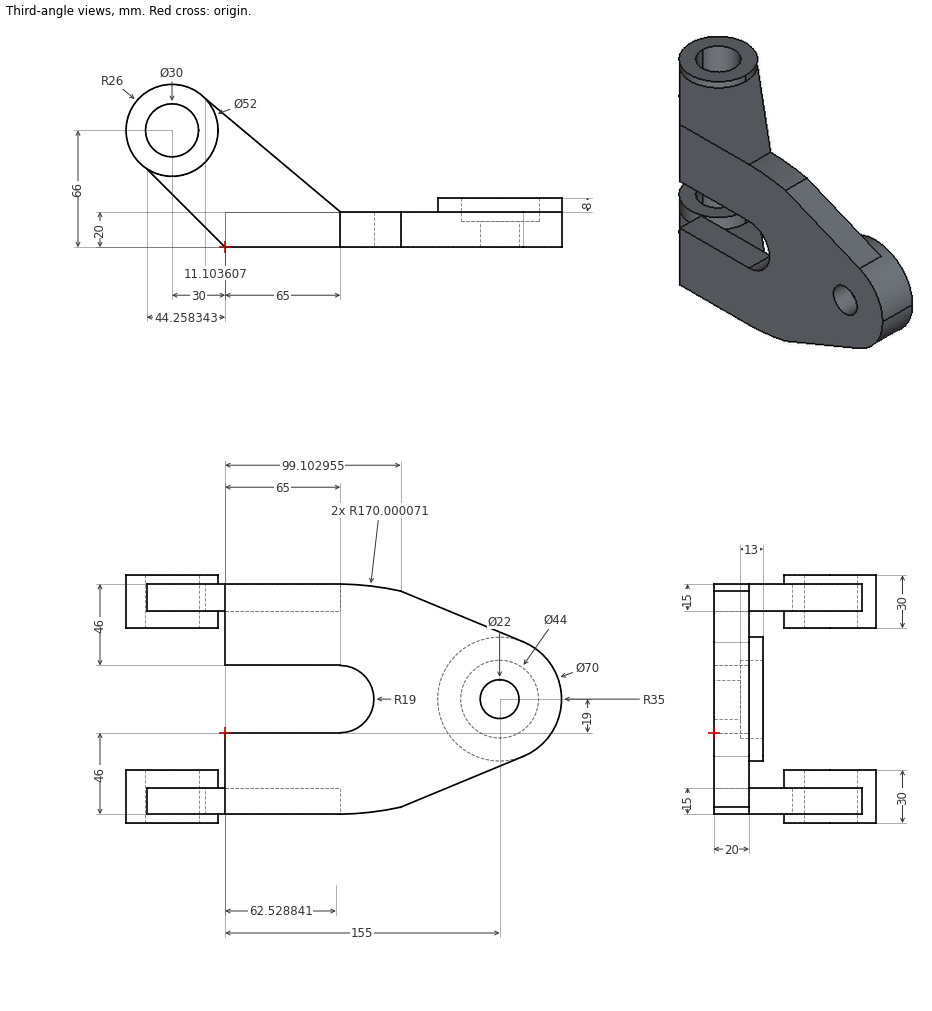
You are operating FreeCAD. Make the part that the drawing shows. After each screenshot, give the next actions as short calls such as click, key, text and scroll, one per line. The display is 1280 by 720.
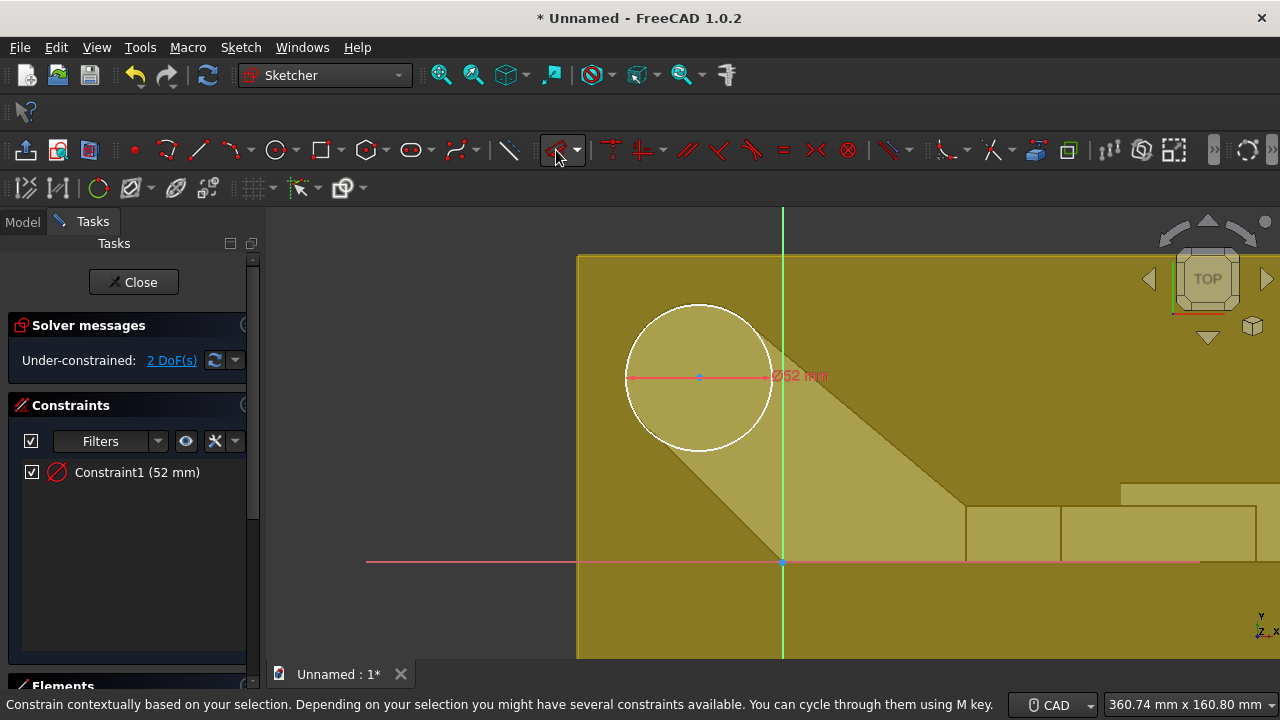
click(699, 378)
click(741, 596)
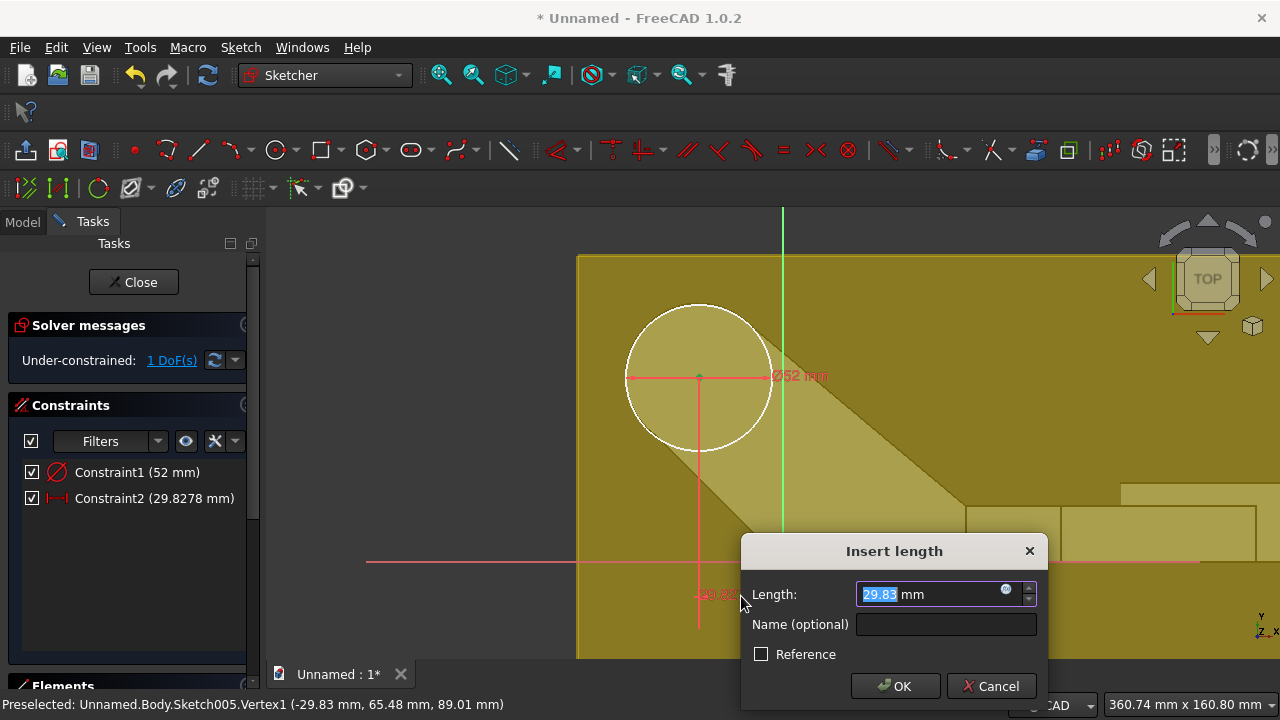
text(30)
key(Return)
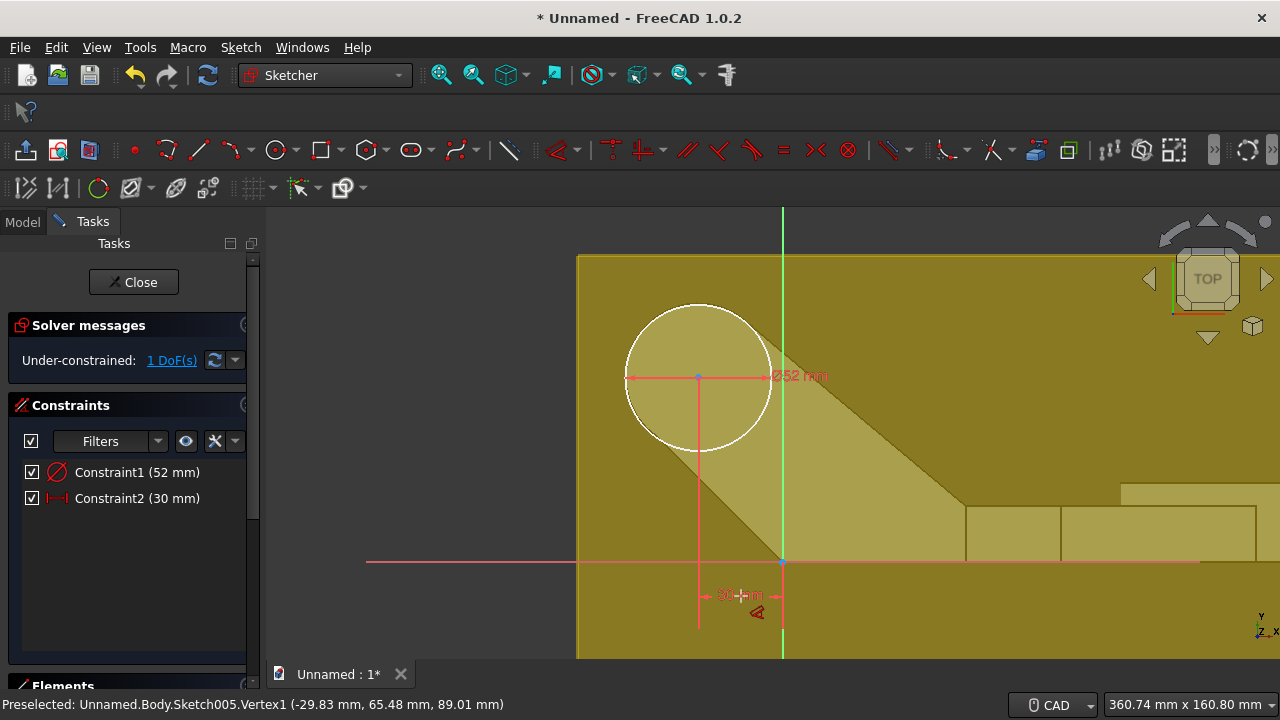
click(699, 378)
click(817, 470)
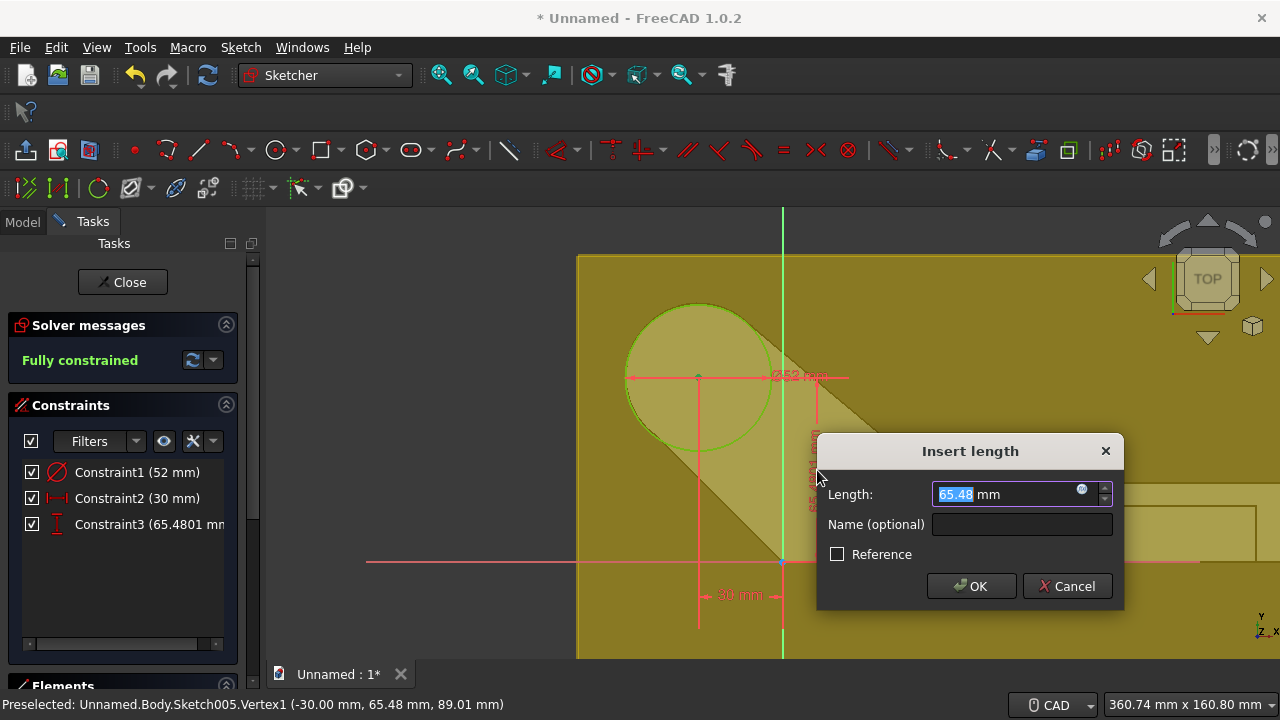
text(66)
key(Return)
key(Escape)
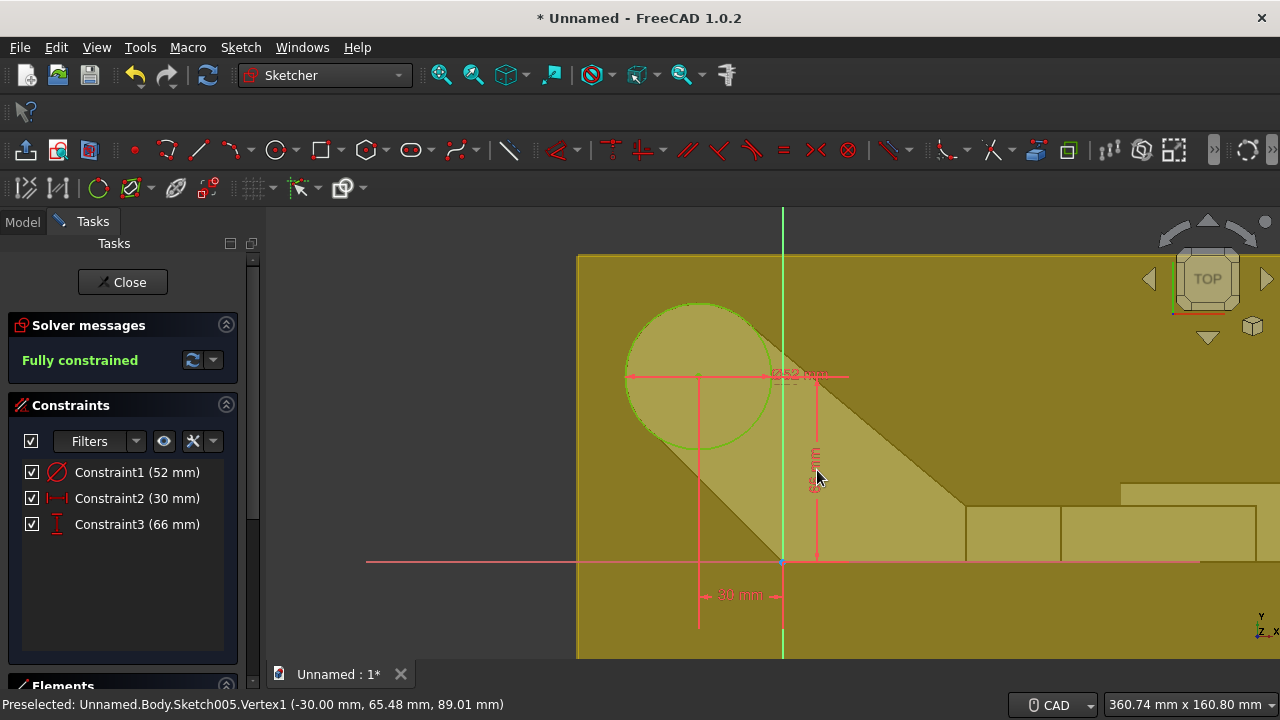
click(123, 282)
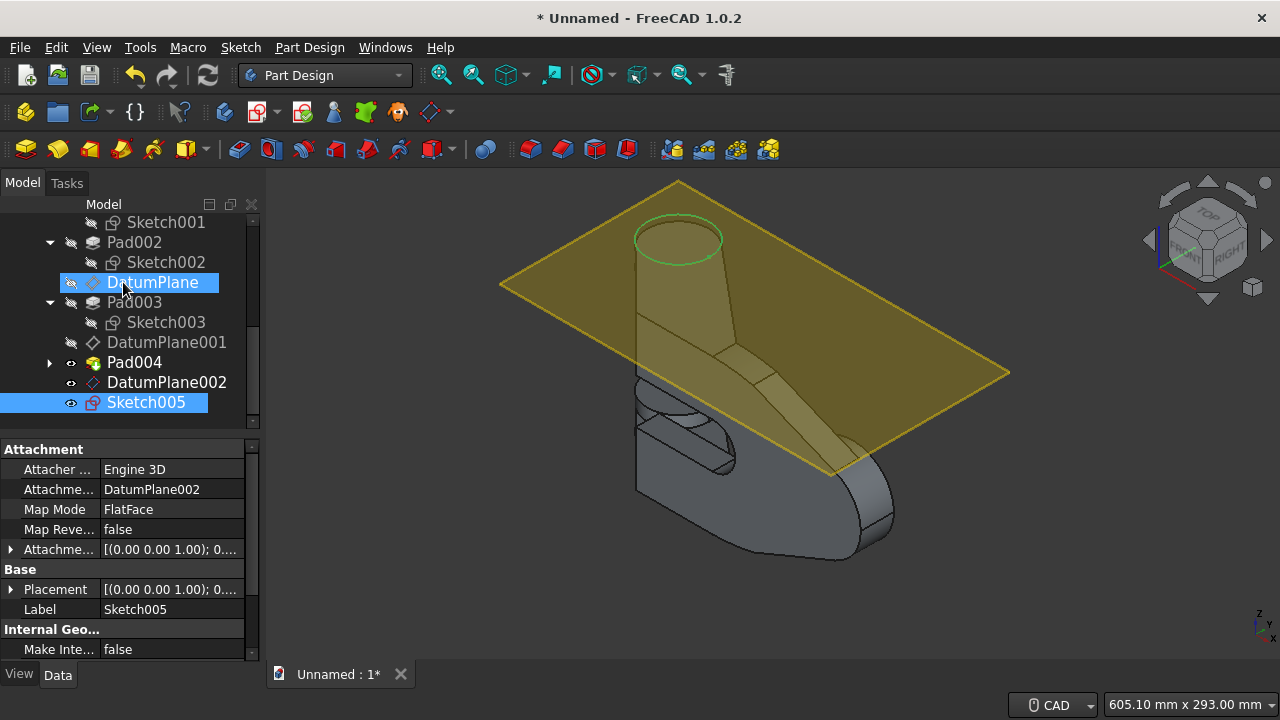
click(26, 150)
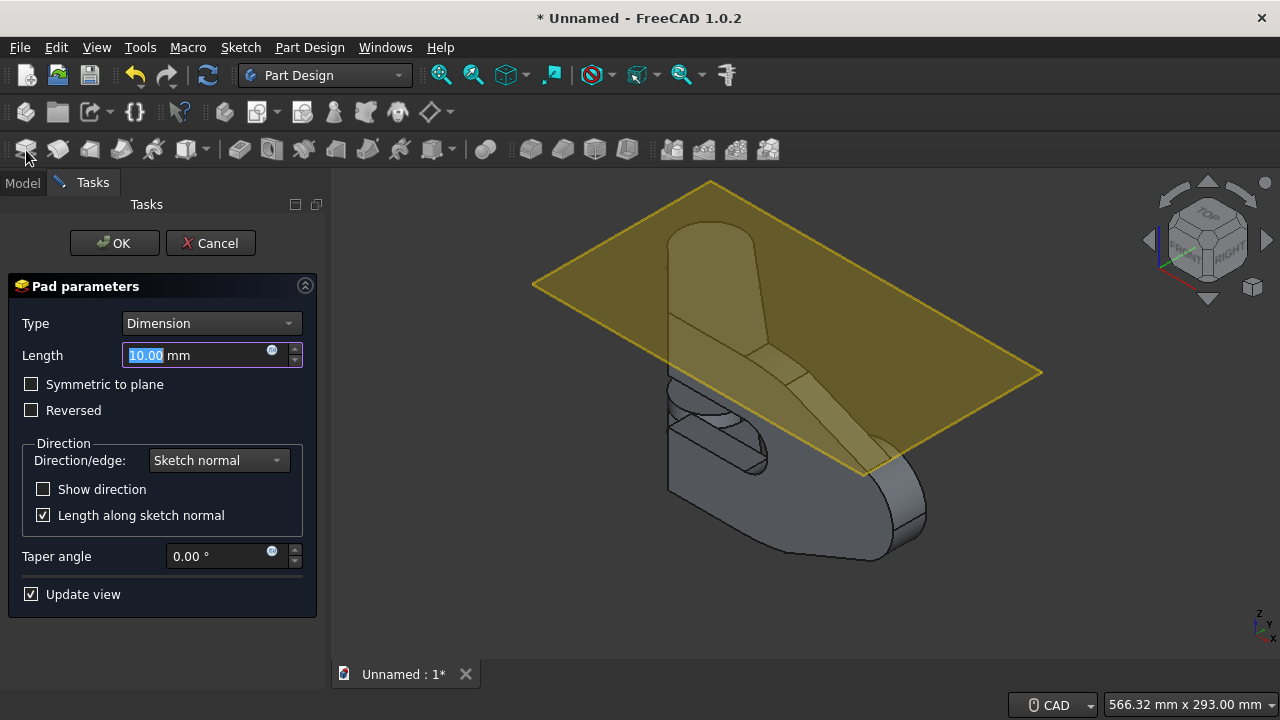
text(30)
key(Tab)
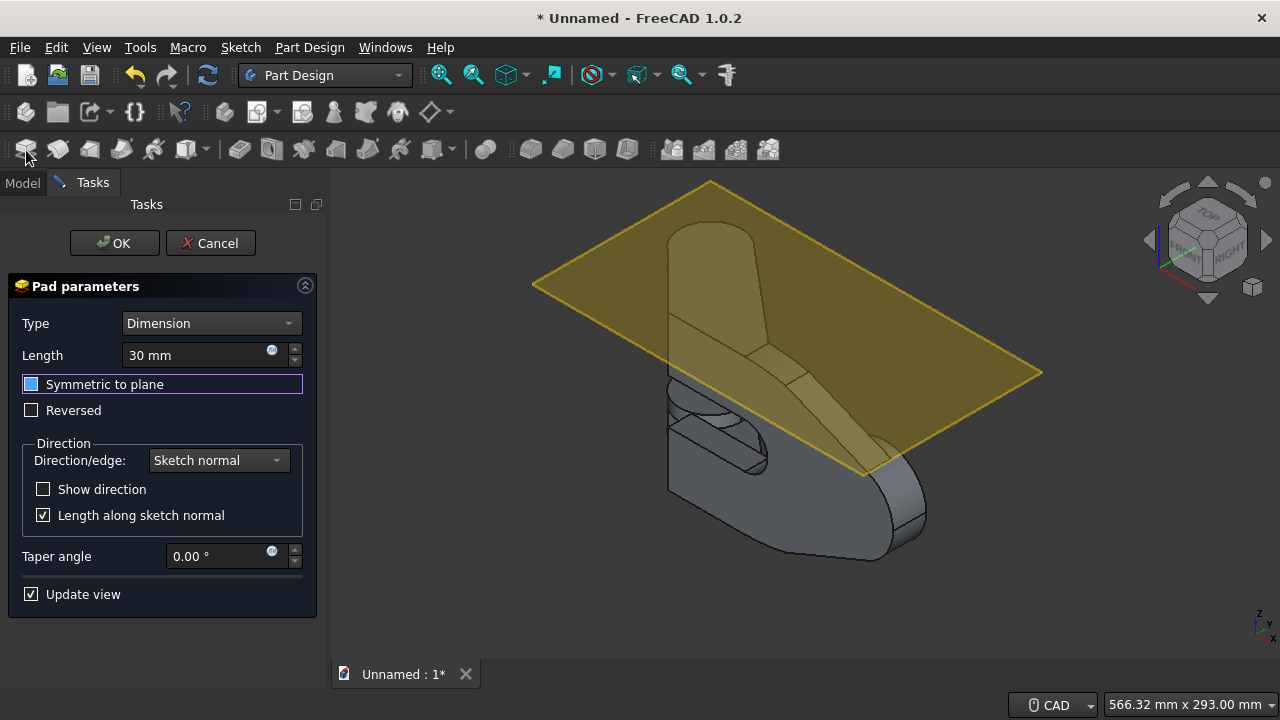
click(30, 410)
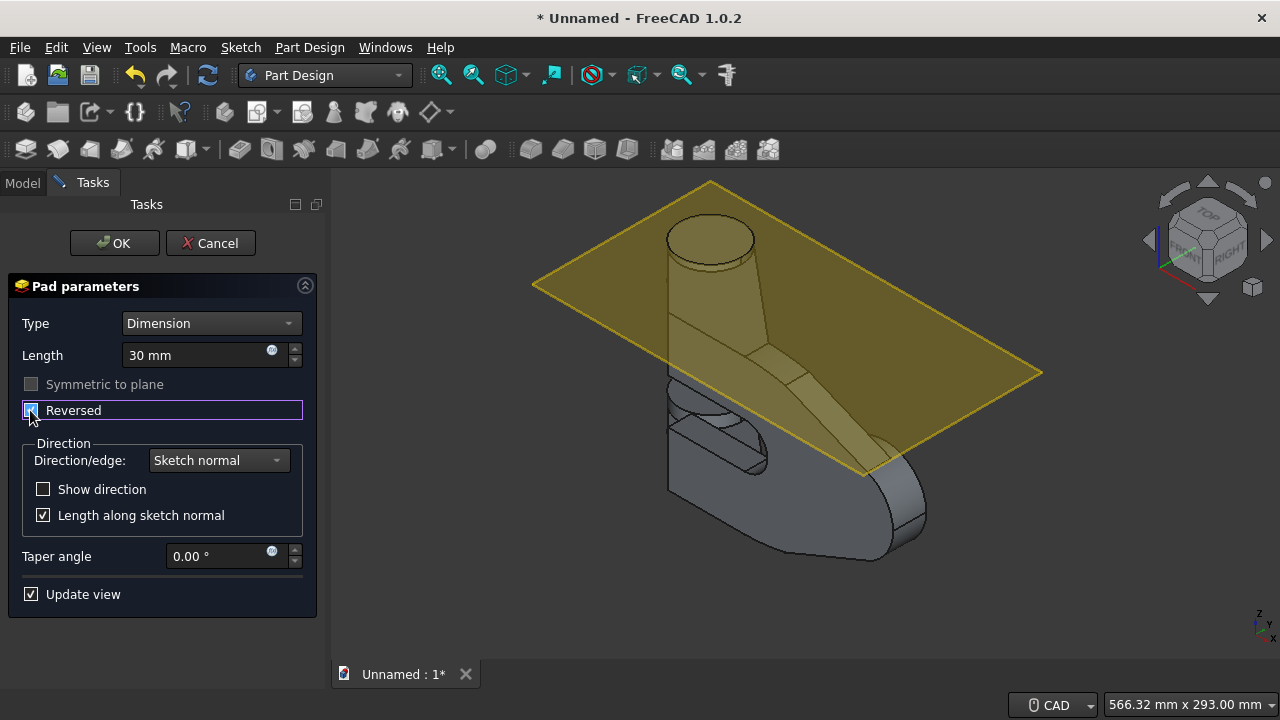
click(115, 243)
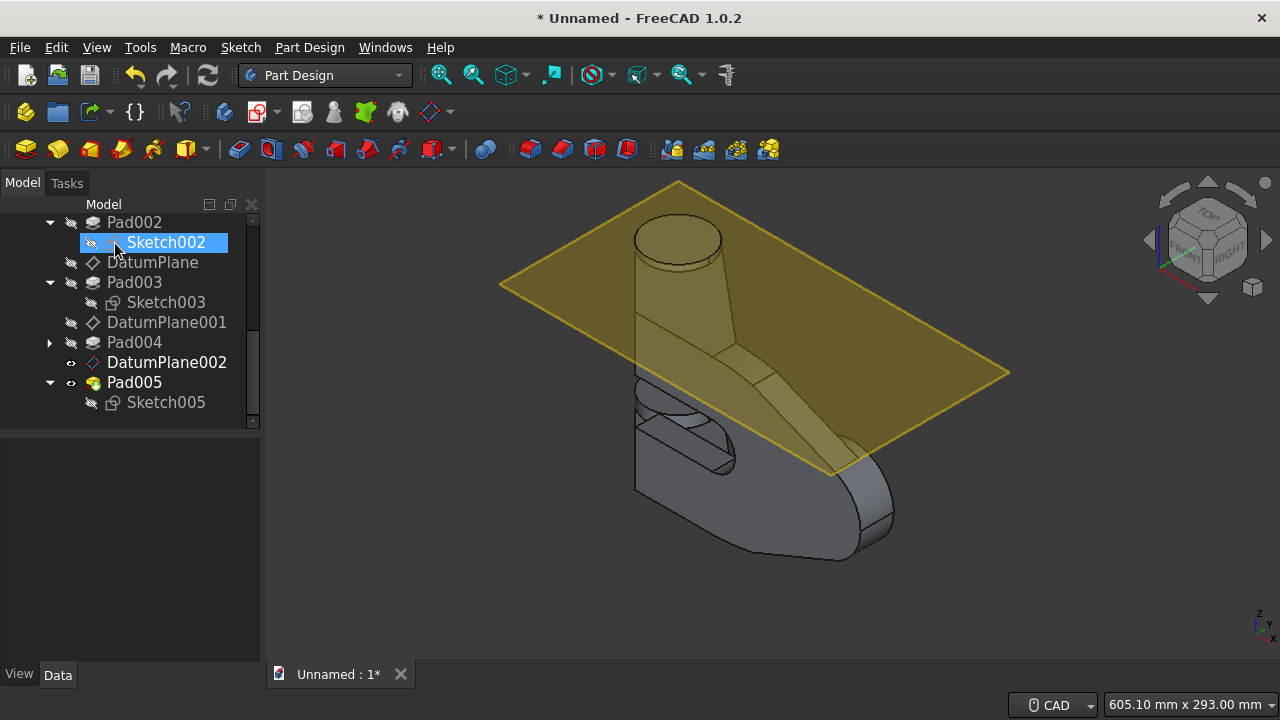
click(116, 363)
key(space)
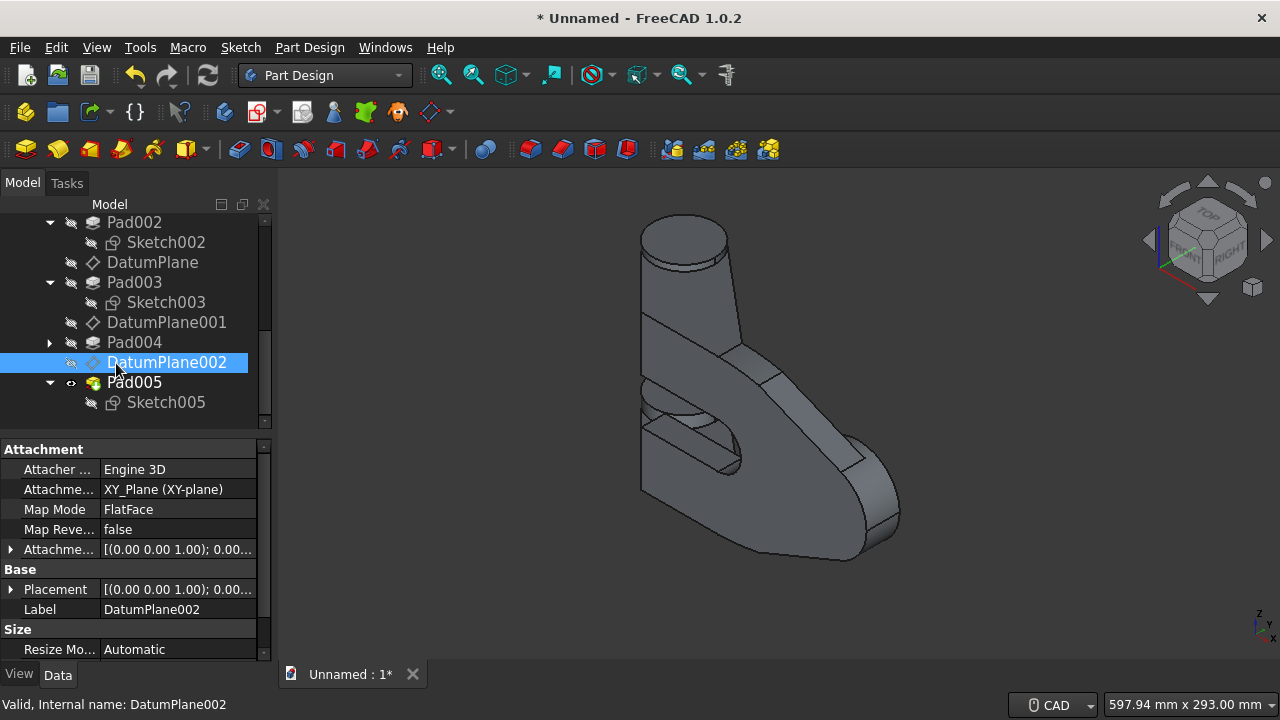
click(684, 239)